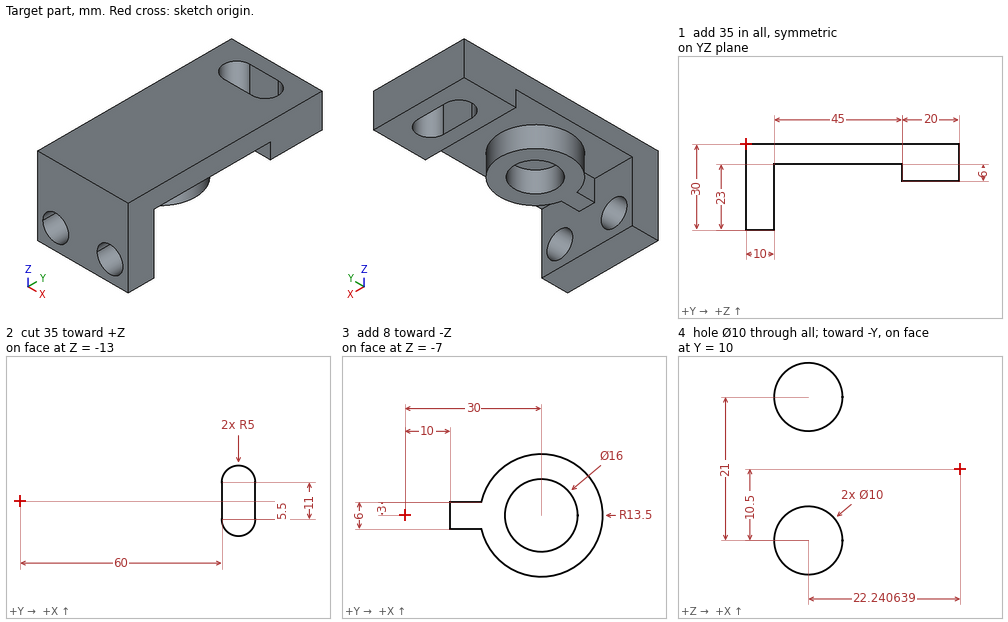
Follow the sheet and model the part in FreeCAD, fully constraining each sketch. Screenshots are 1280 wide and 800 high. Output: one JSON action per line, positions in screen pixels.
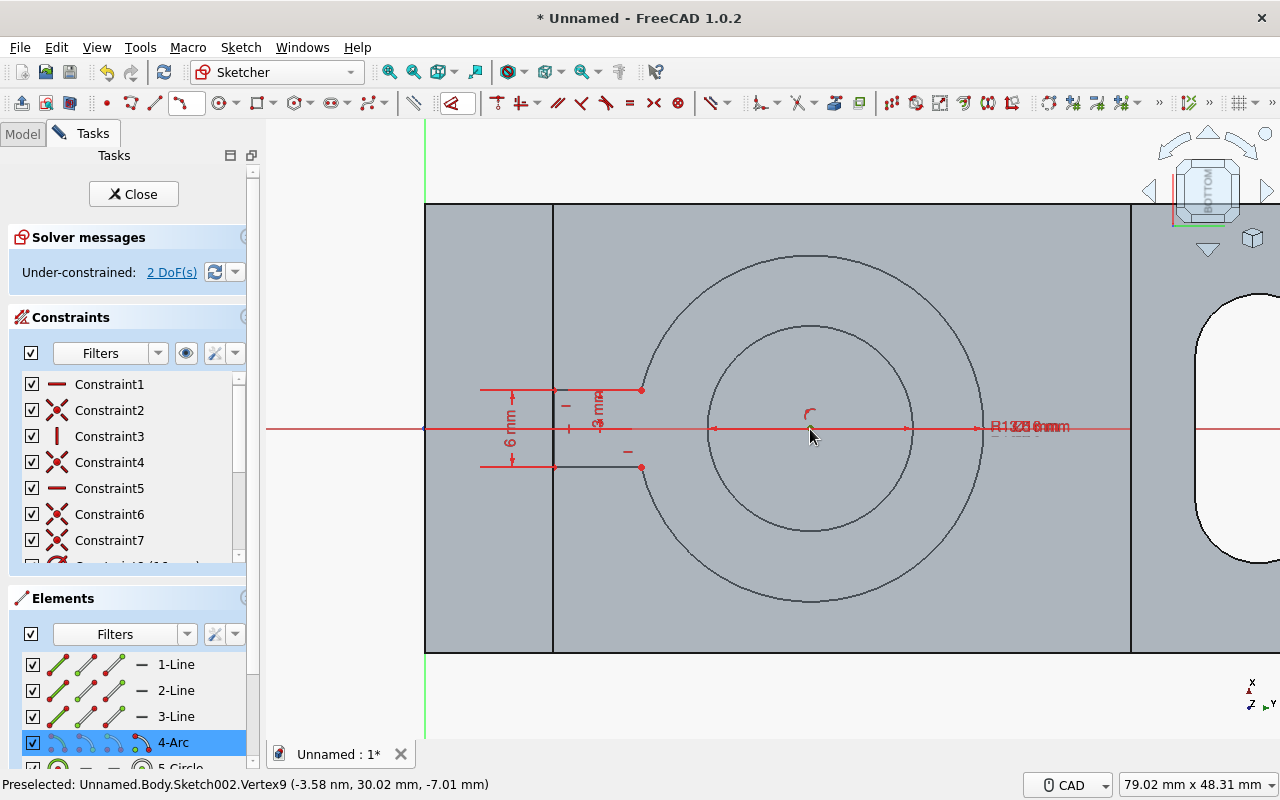
{"action": "key", "text": "l"}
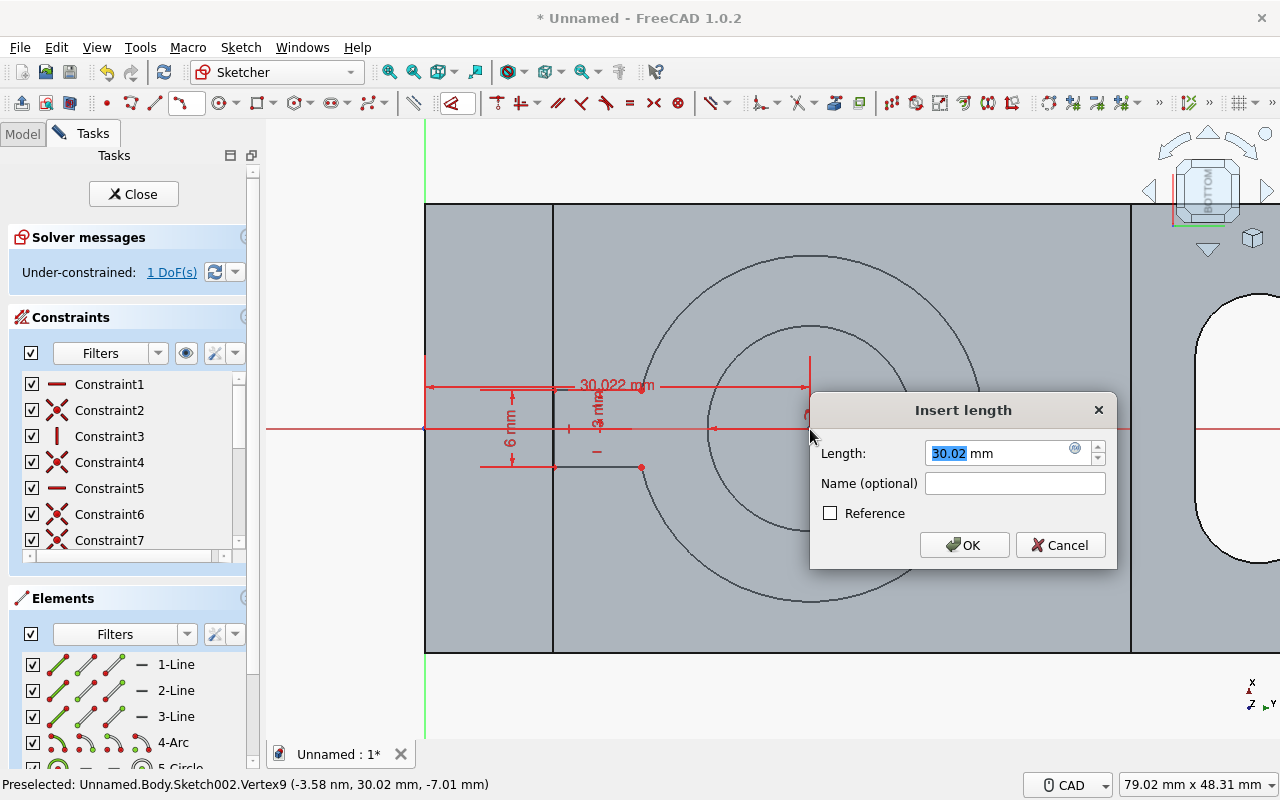
{"action": "type", "text": "30"}
{"action": "key", "text": "Return"}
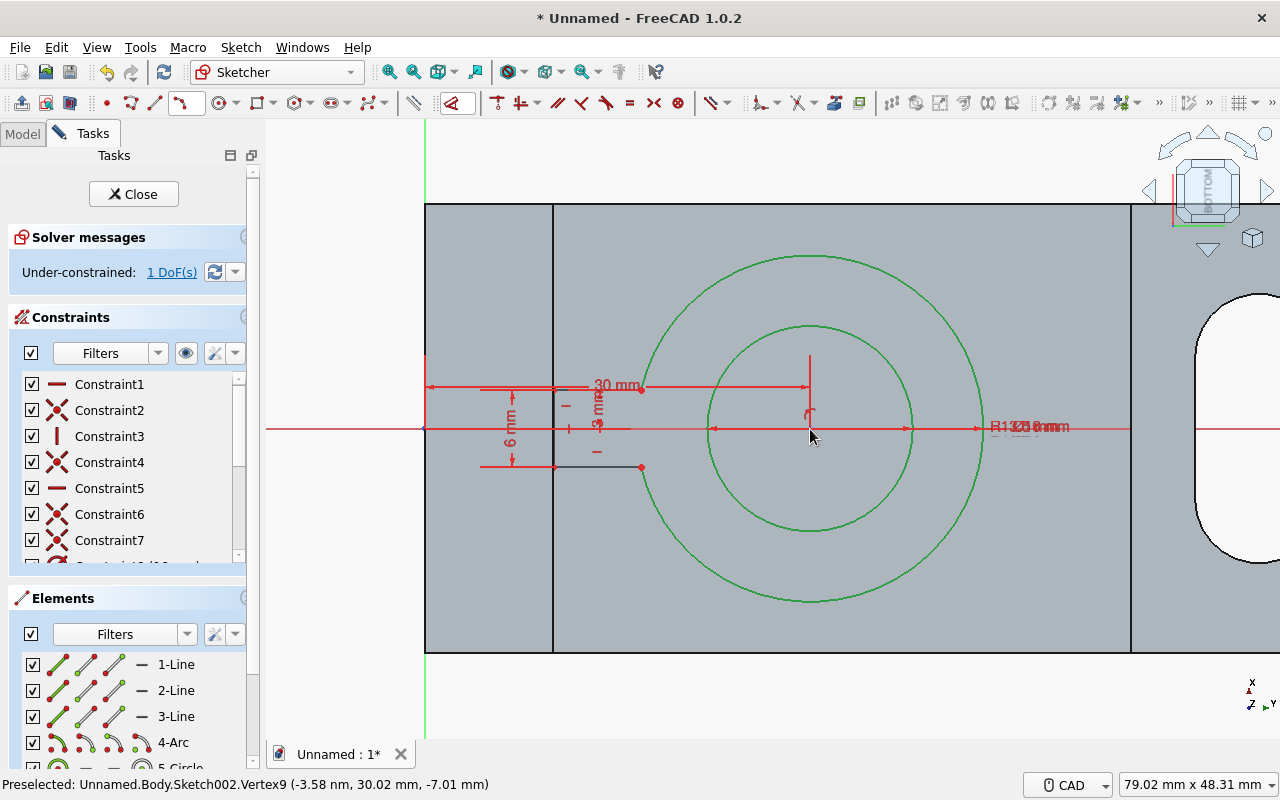
{"action": "left_click", "coordinate": [554, 390]}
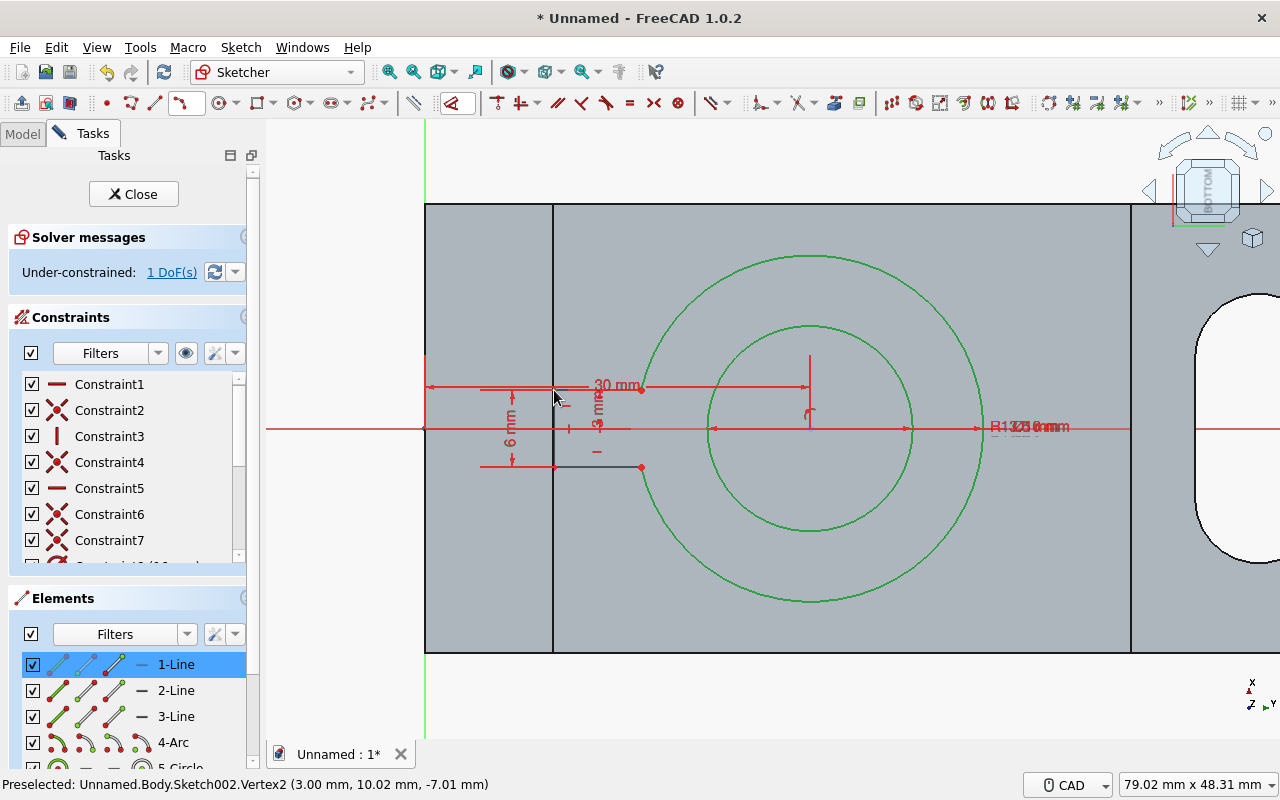
{"action": "key", "text": "l"}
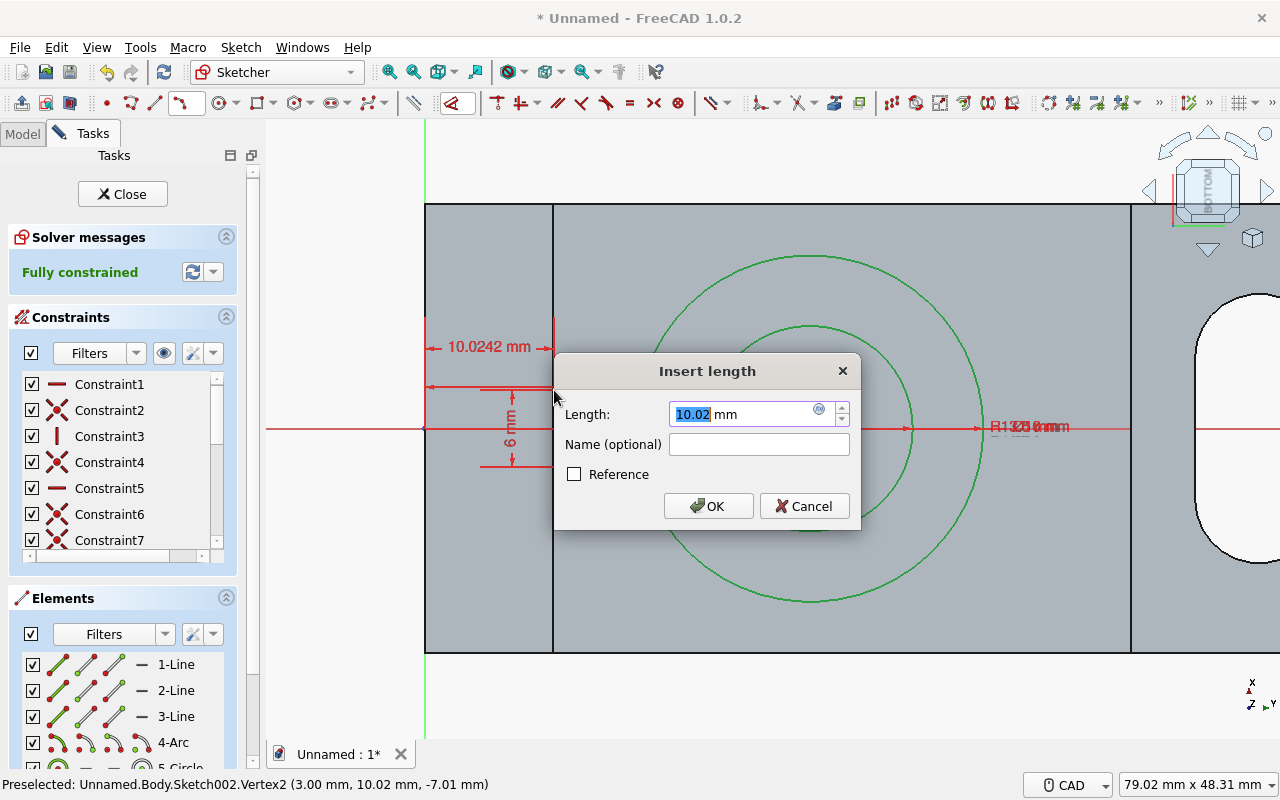
{"action": "type", "text": "10"}
{"action": "key", "text": "Return"}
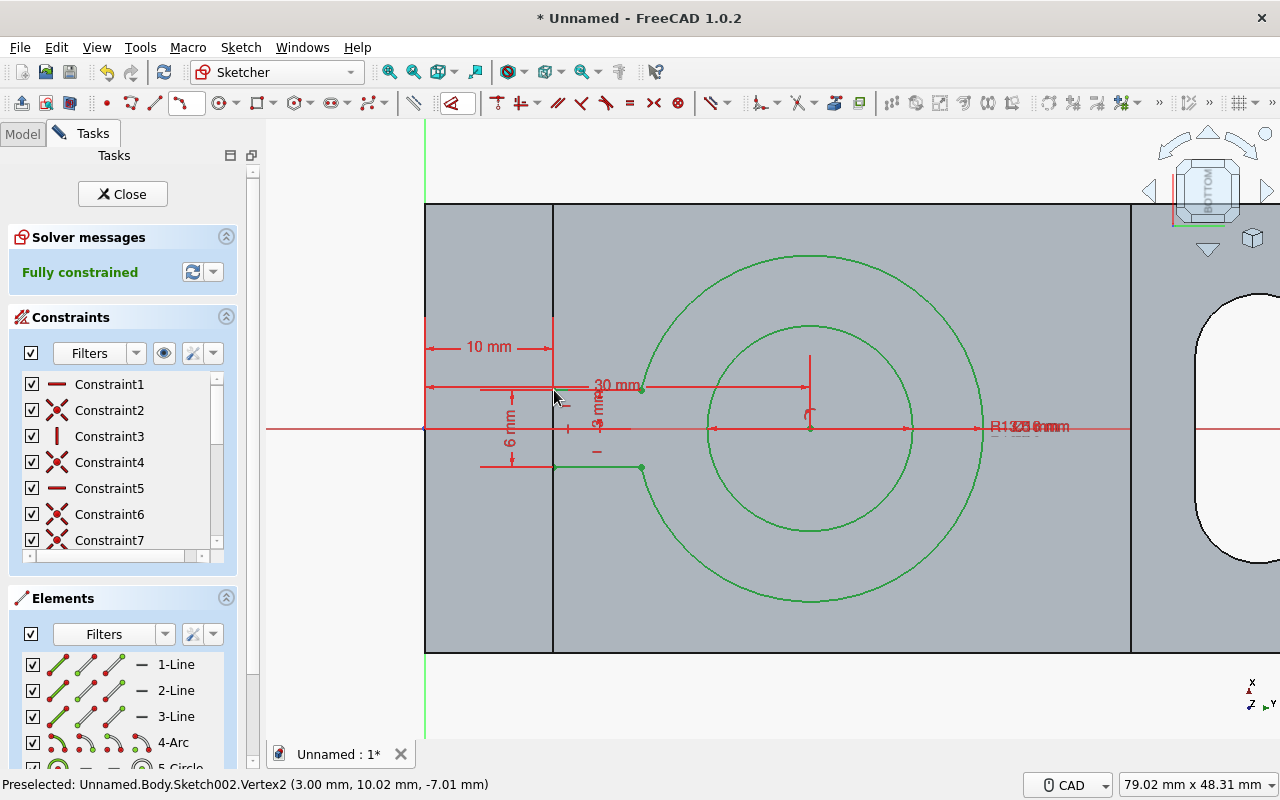
{"action": "left_click", "coordinate": [123, 194]}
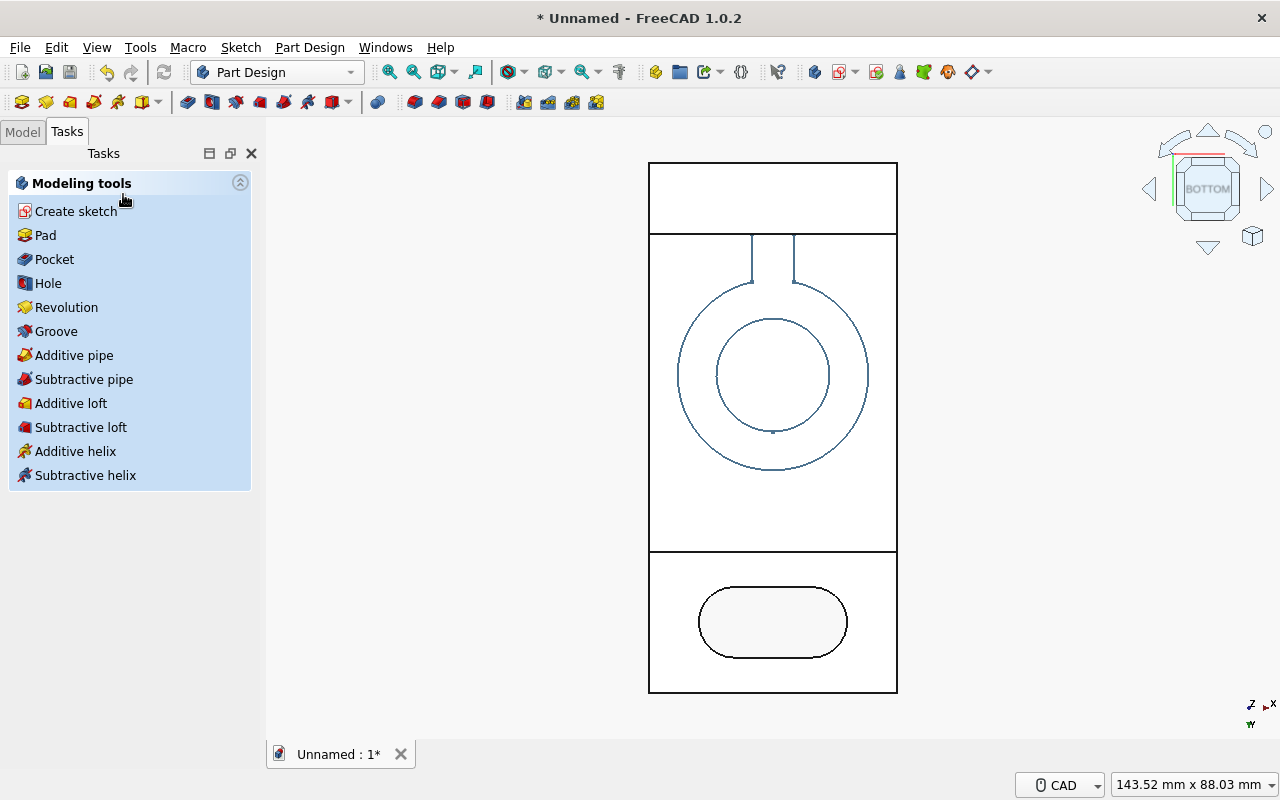
{"action": "left_click", "coordinate": [22, 102]}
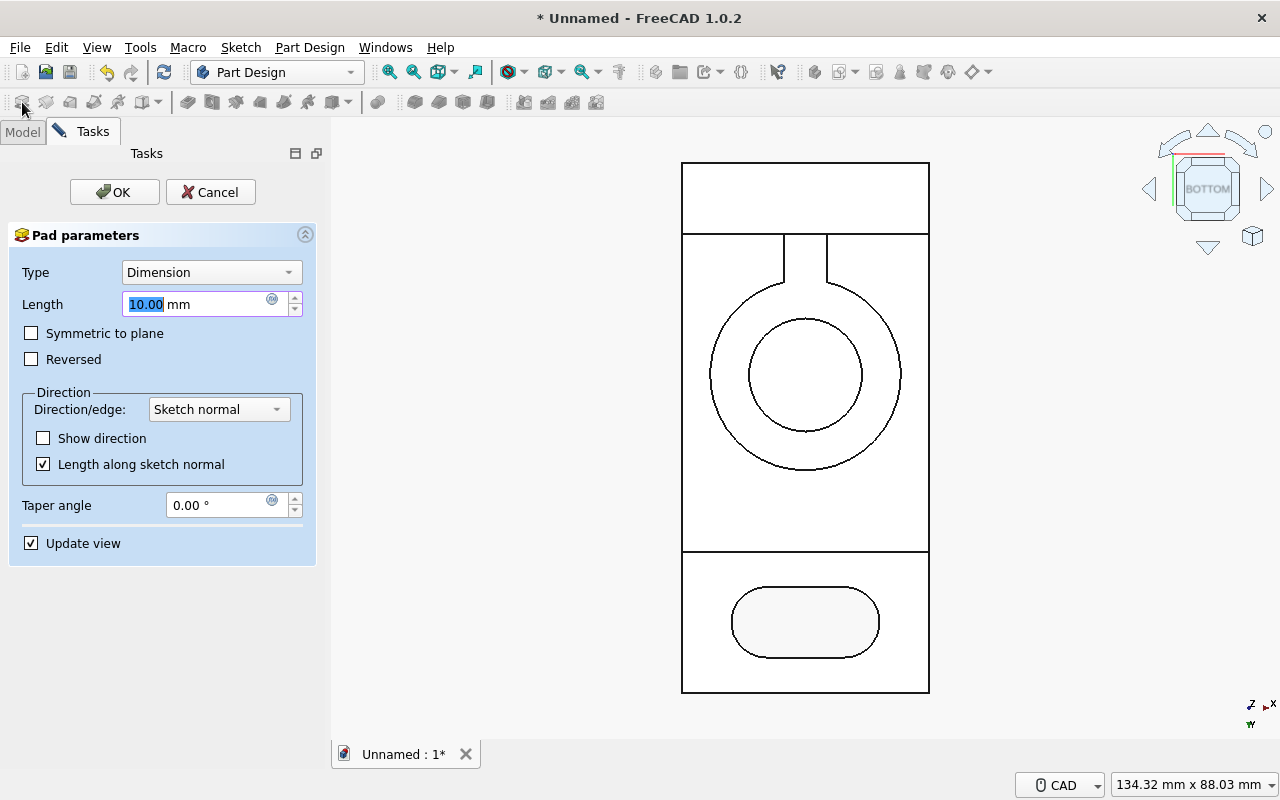
{"action": "type", "text": "8"}
{"action": "key", "text": "Tab"}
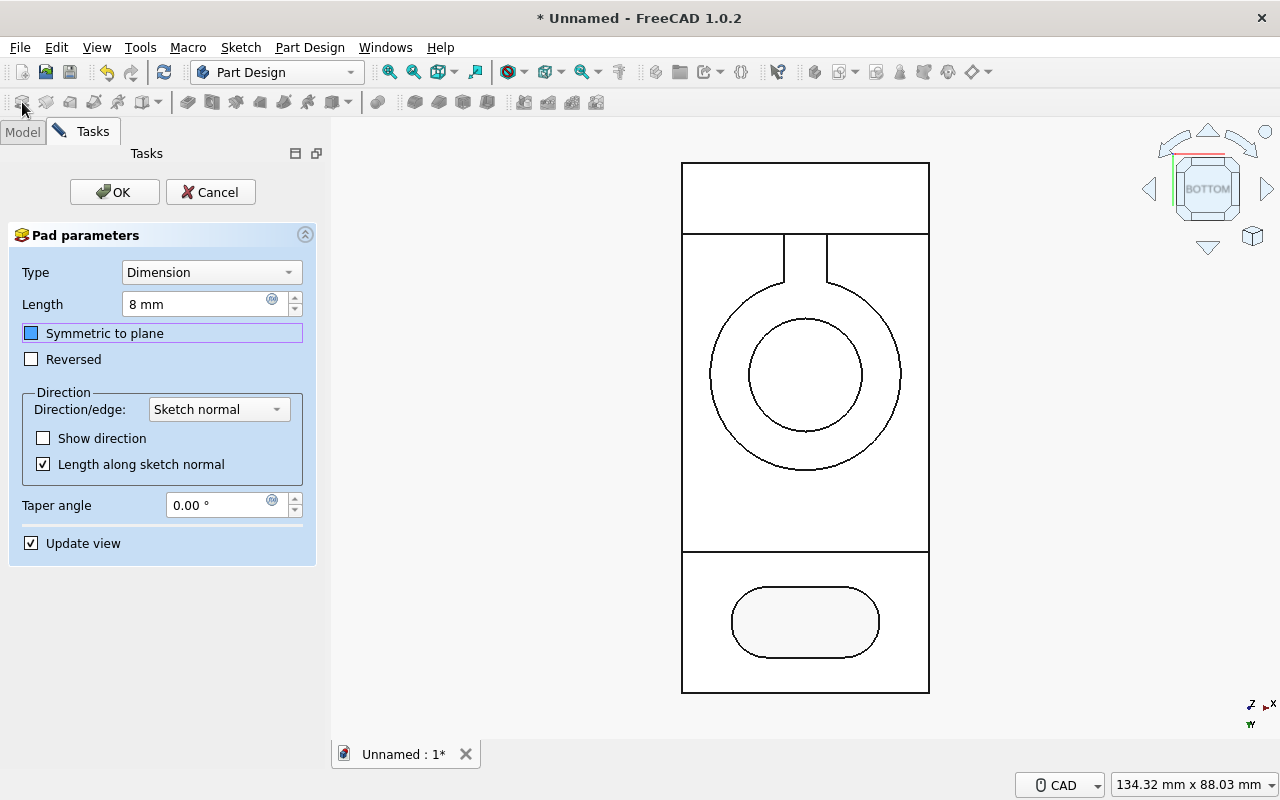
{"action": "left_click", "coordinate": [115, 192]}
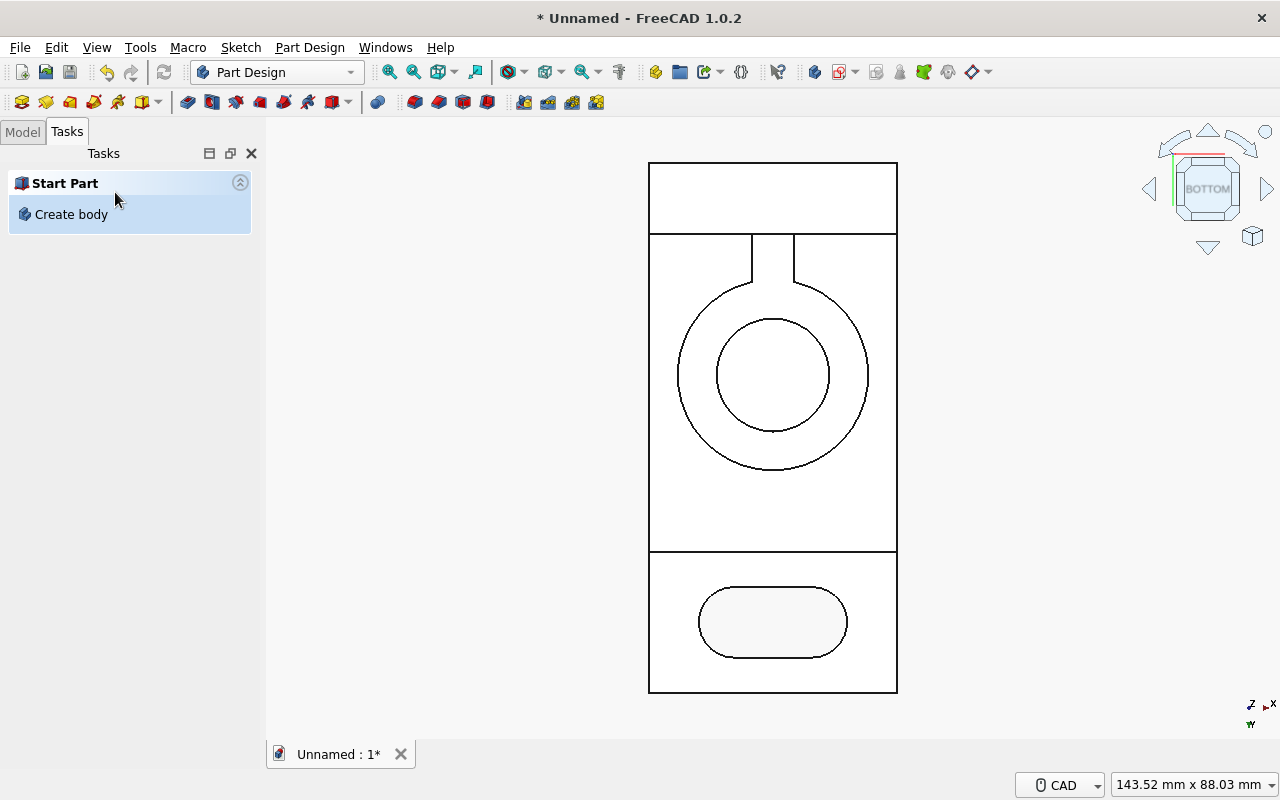
{"action": "key", "text": "4"}